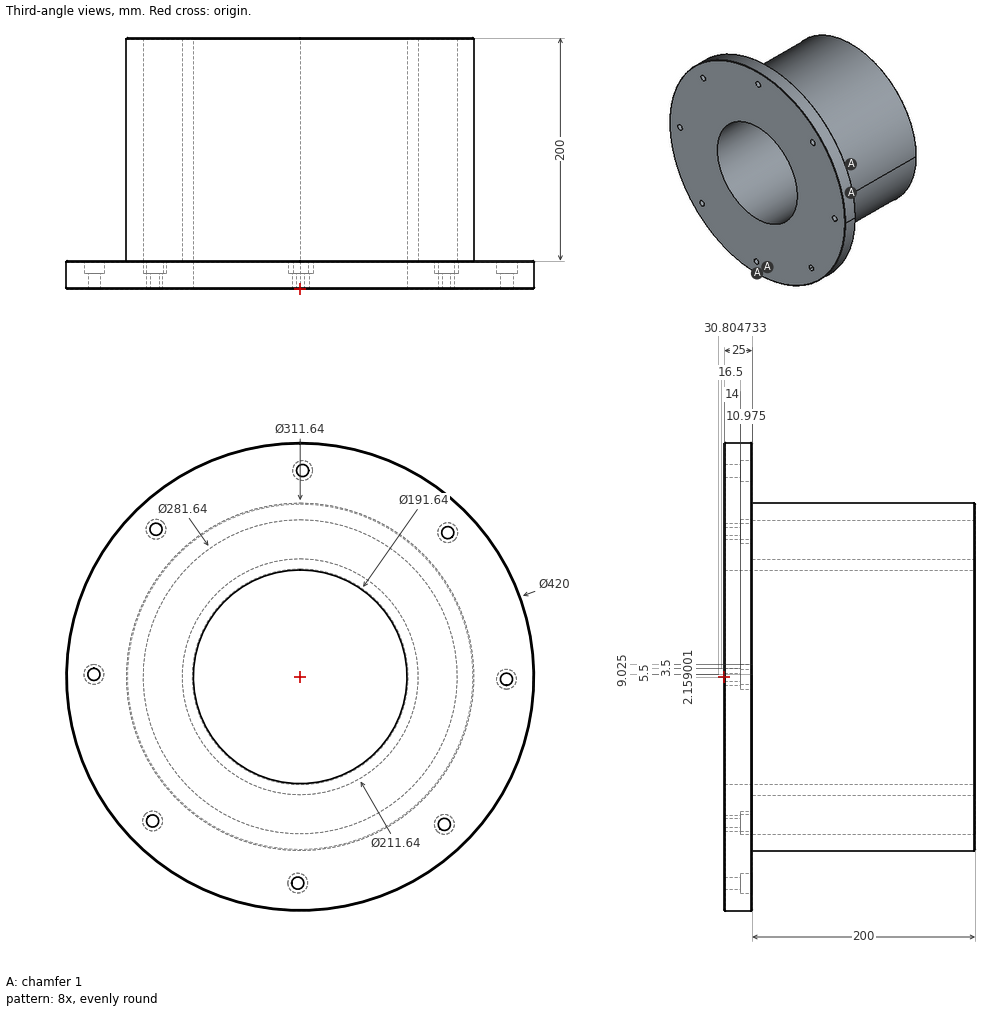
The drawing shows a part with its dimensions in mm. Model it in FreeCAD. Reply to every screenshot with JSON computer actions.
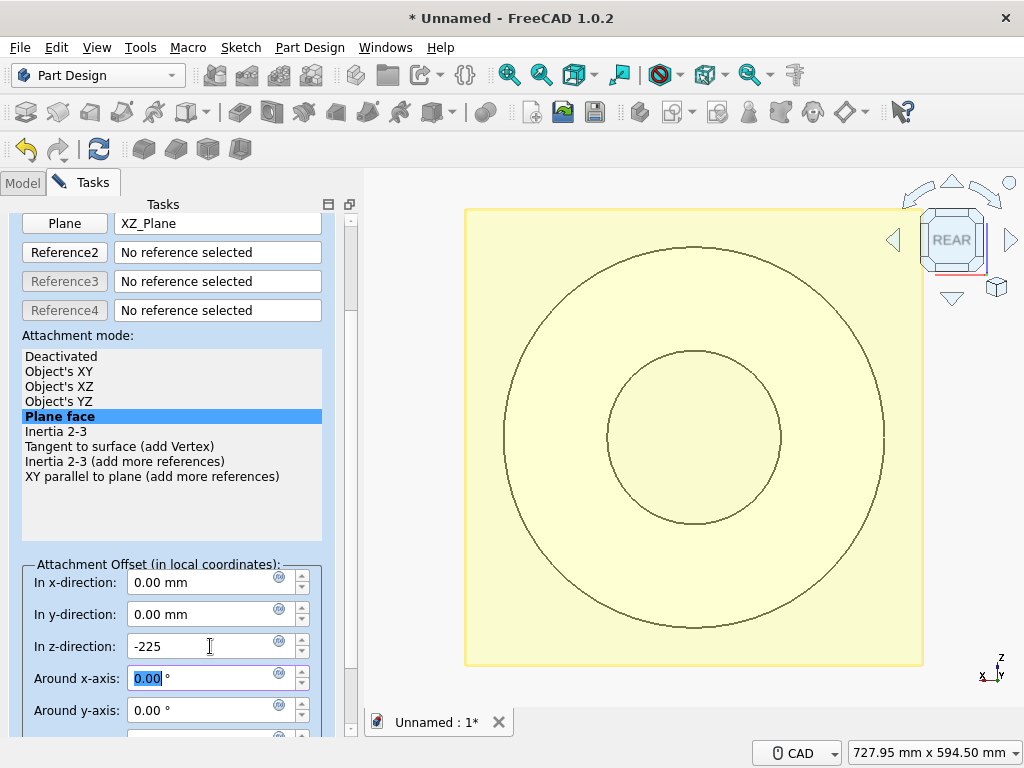
{"action": "scroll", "coordinate": [351, 475], "scroll_direction": "up", "scroll_amount": 3}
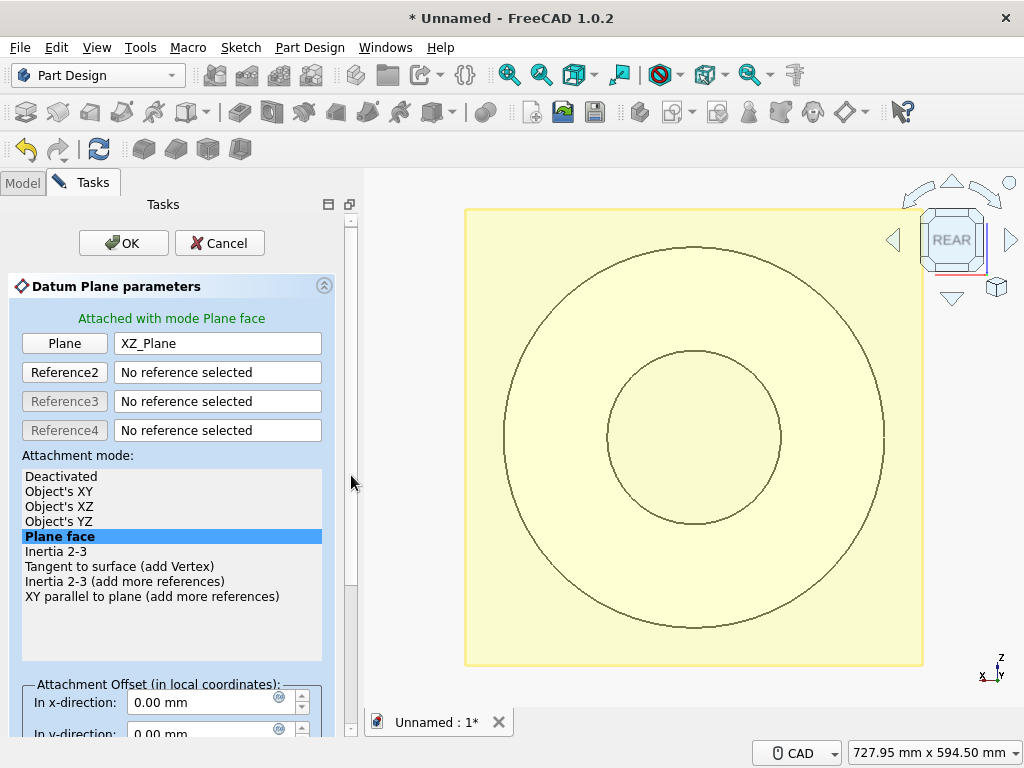
{"action": "left_click", "coordinate": [124, 243]}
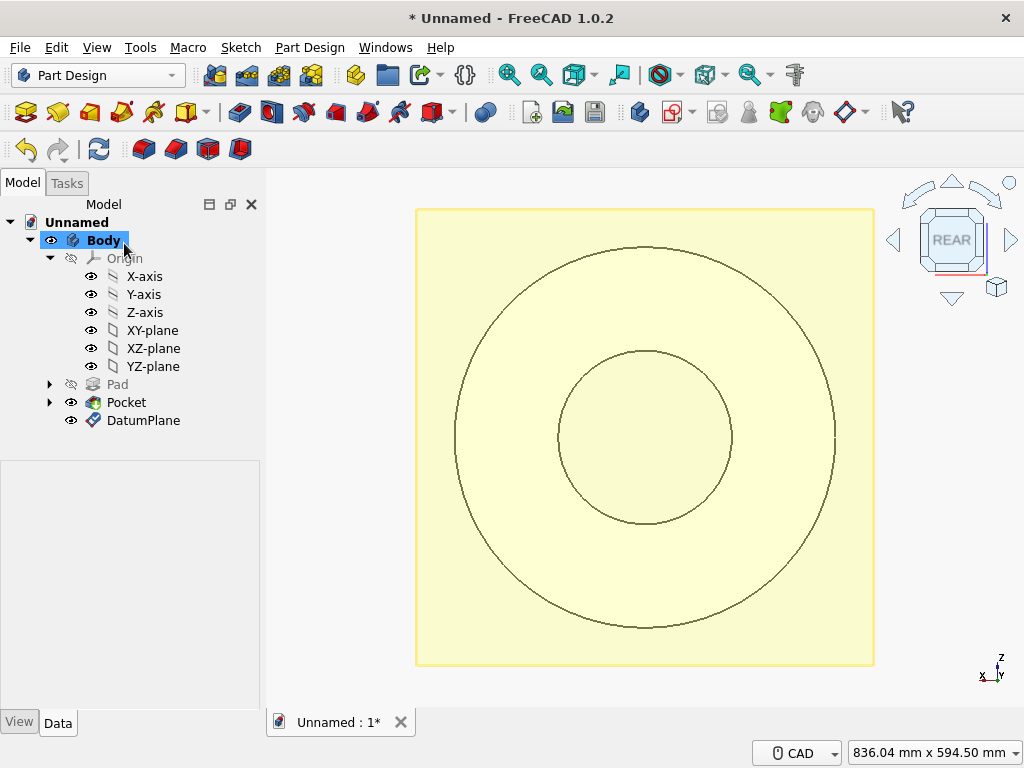
{"action": "left_click", "coordinate": [116, 420]}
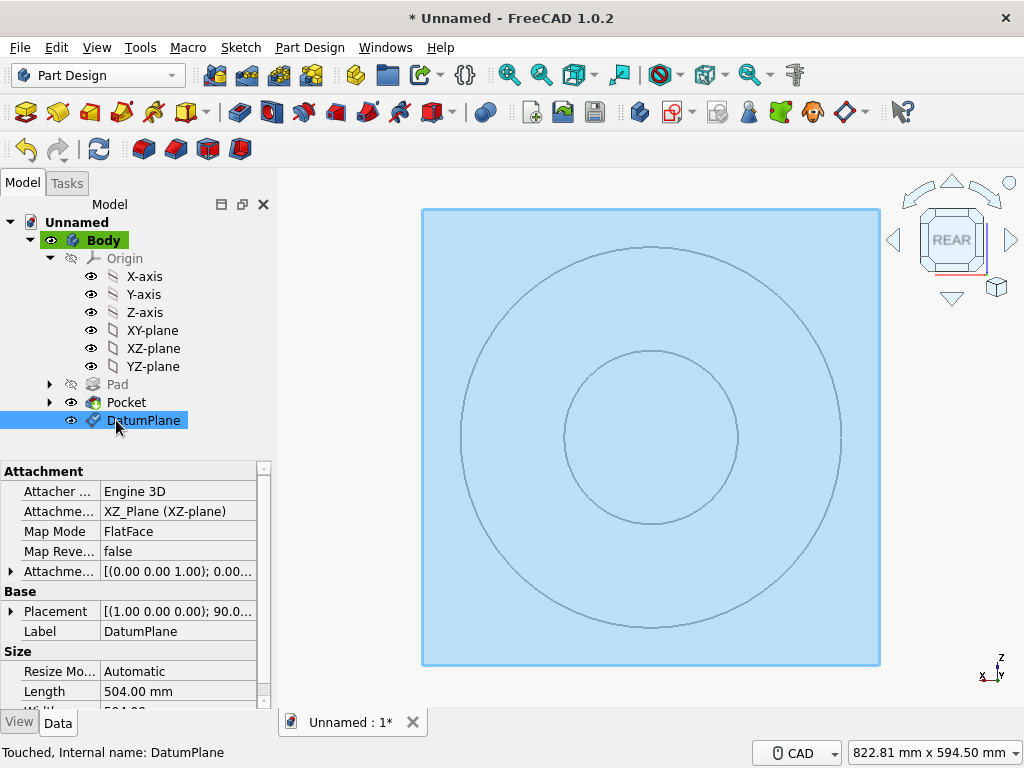
{"action": "left_click", "coordinate": [672, 112]}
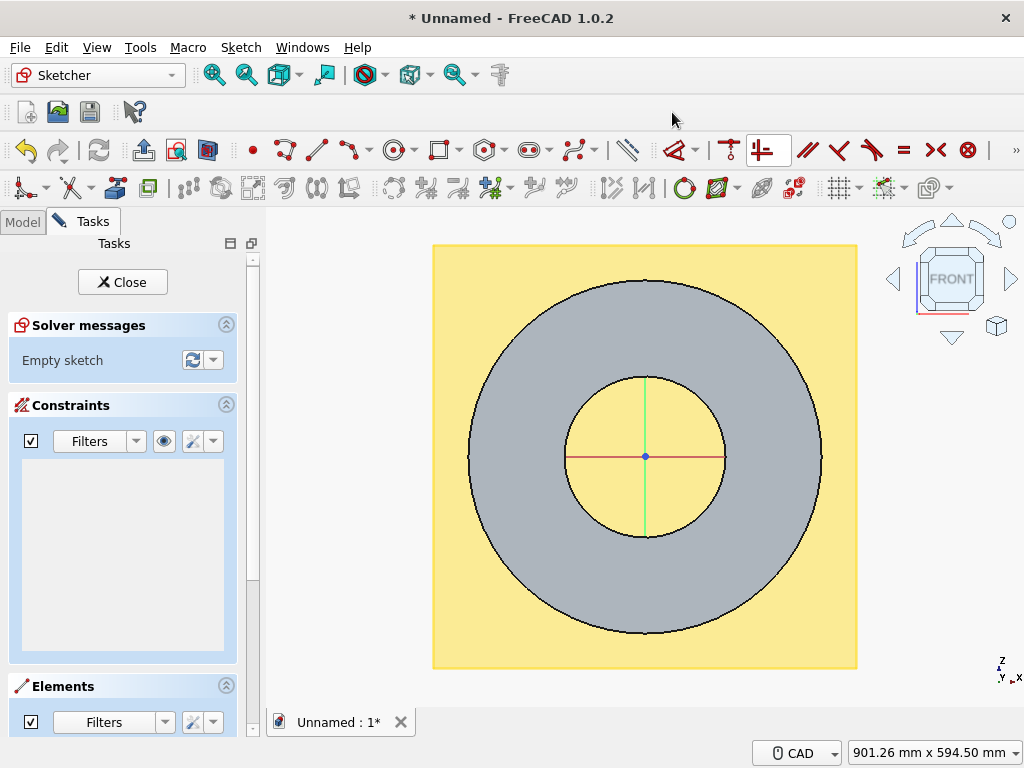
{"action": "left_click", "coordinate": [208, 150]}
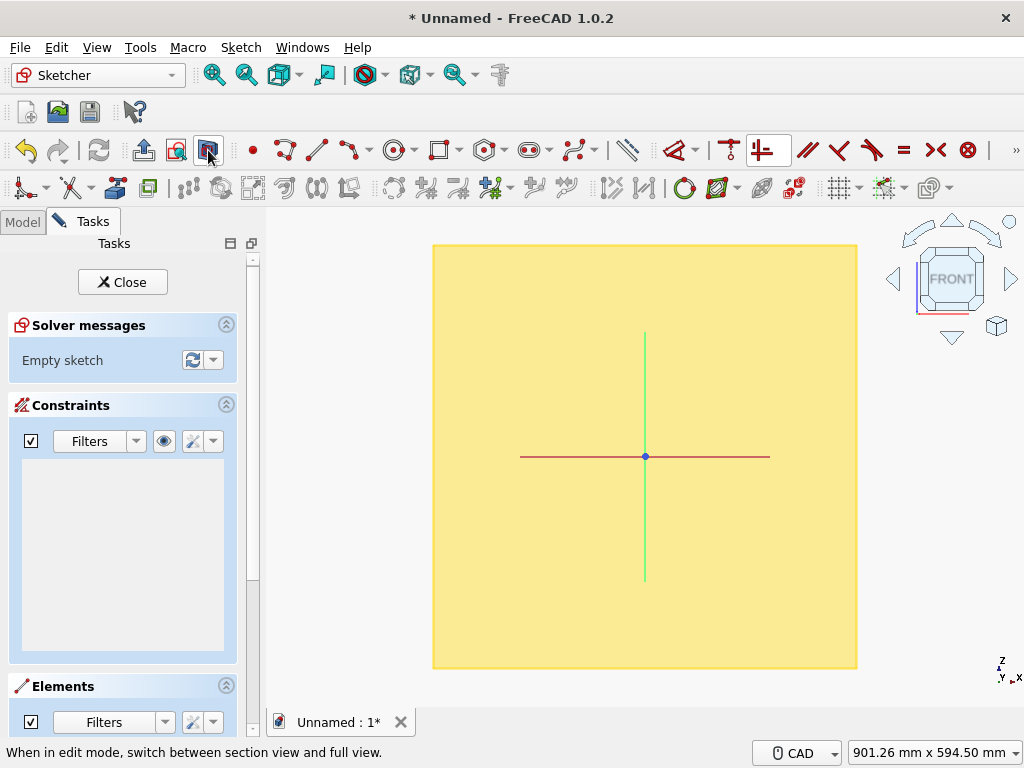
{"action": "left_click", "coordinate": [394, 150]}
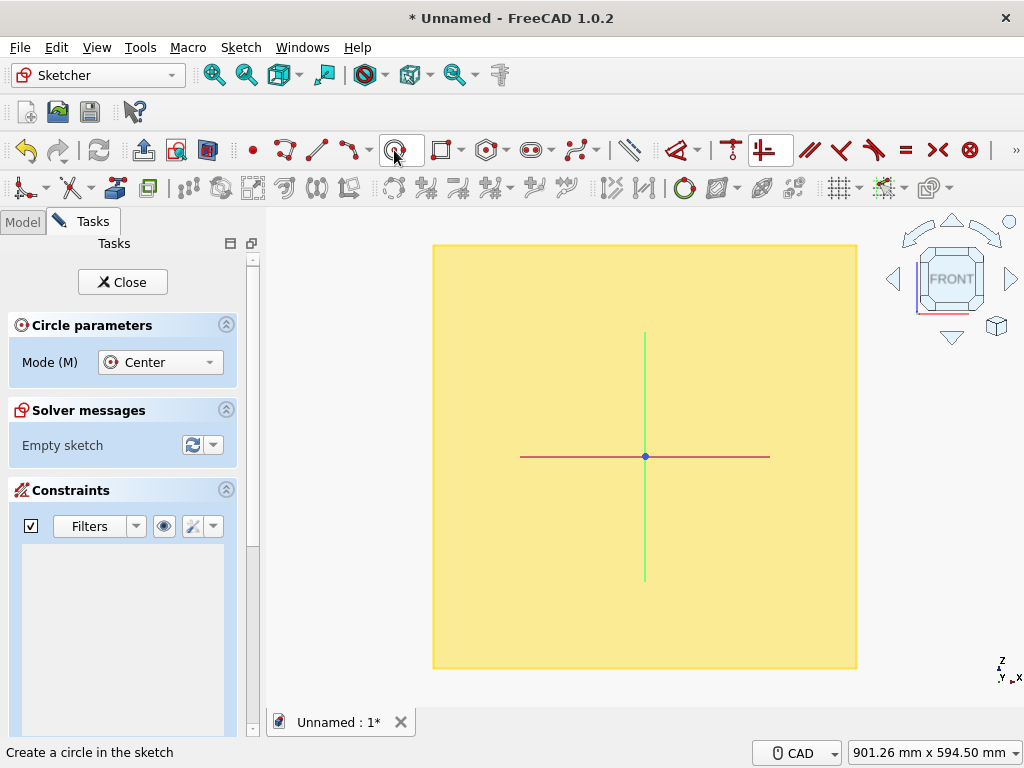
{"action": "left_click", "coordinate": [645, 457]}
{"action": "left_click", "coordinate": [738, 364]}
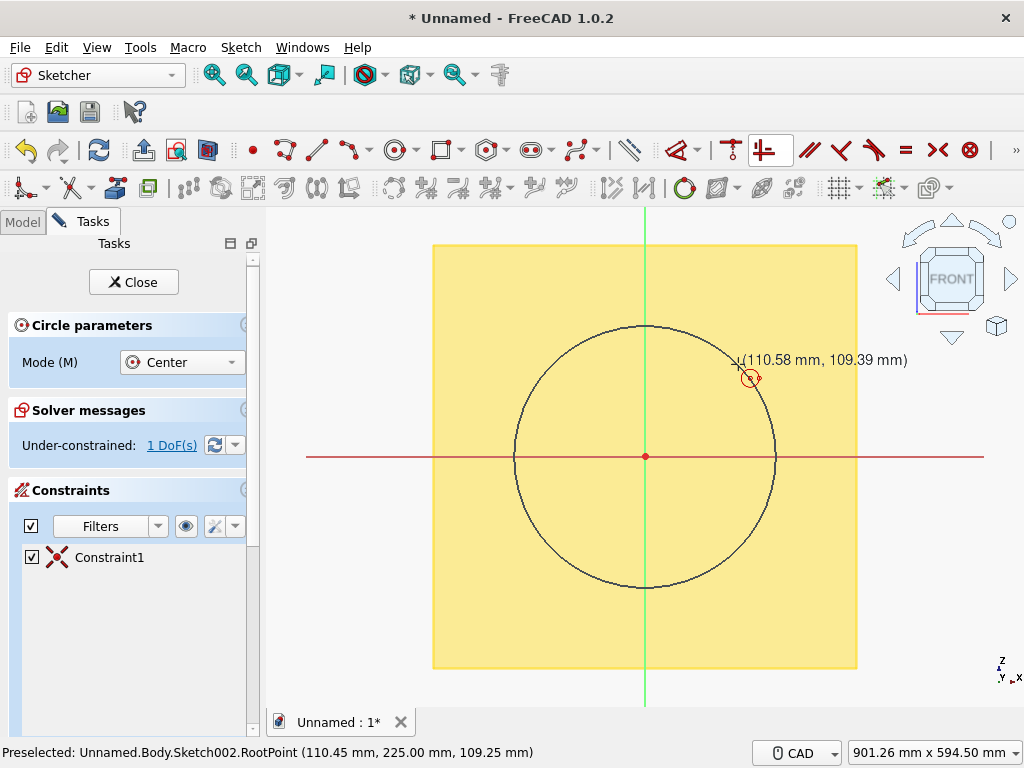
{"action": "left_click", "coordinate": [645, 457]}
{"action": "left_click", "coordinate": [702, 400]}
{"action": "key", "text": "Escape"}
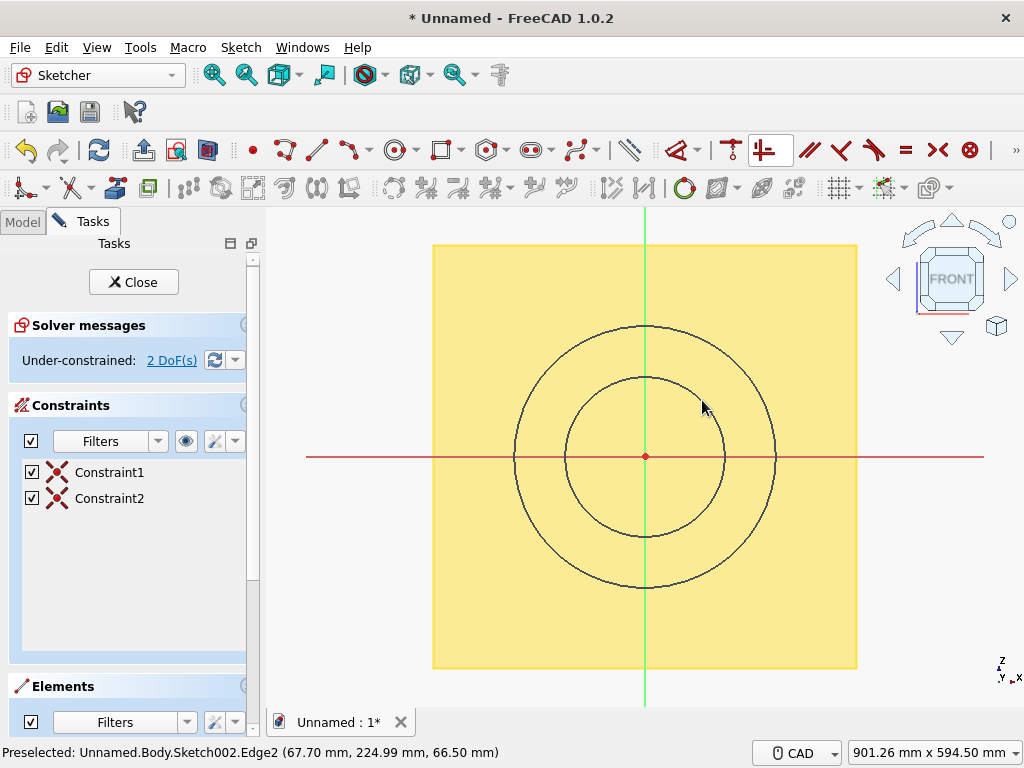
{"action": "key", "text": "d"}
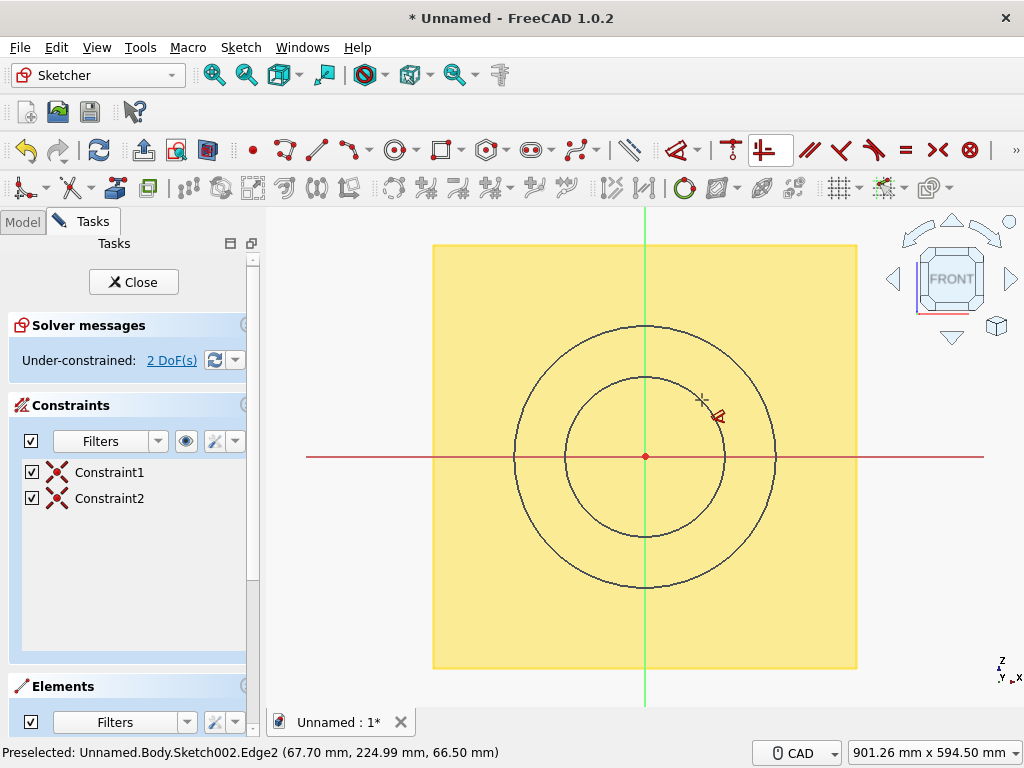
{"action": "left_click", "coordinate": [737, 364]}
{"action": "left_click", "coordinate": [760, 341]}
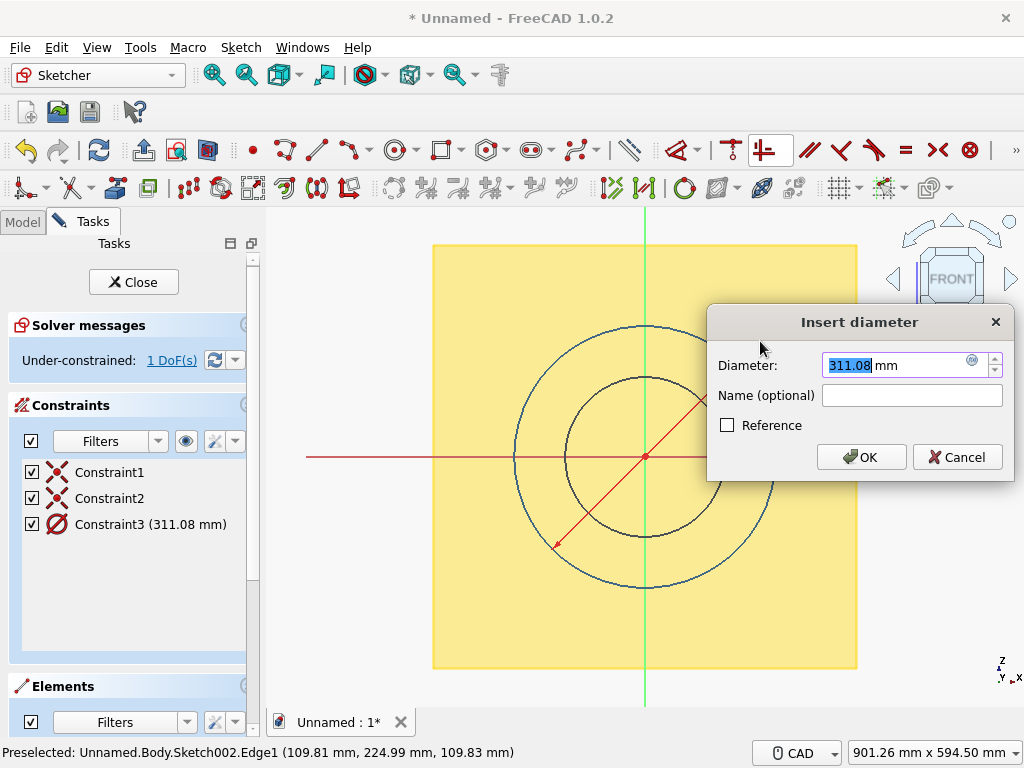
{"action": "type", "text": "311.64"}
{"action": "key", "text": "Return"}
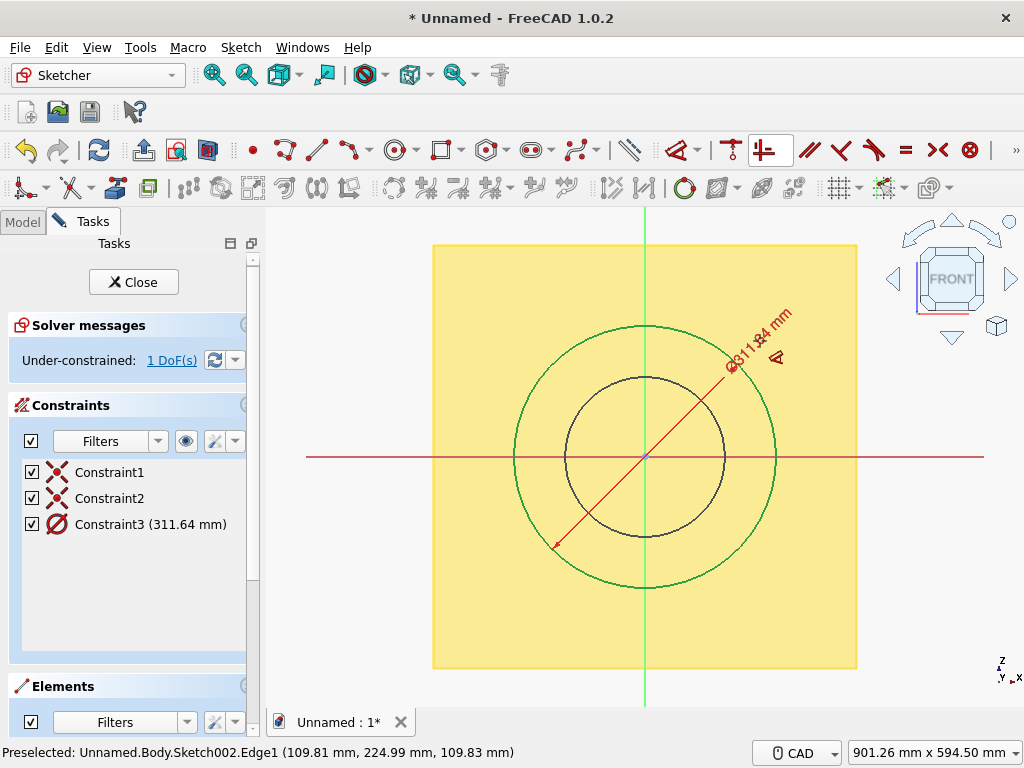
{"action": "left_click", "coordinate": [701, 400]}
{"action": "left_click", "coordinate": [723, 377]}